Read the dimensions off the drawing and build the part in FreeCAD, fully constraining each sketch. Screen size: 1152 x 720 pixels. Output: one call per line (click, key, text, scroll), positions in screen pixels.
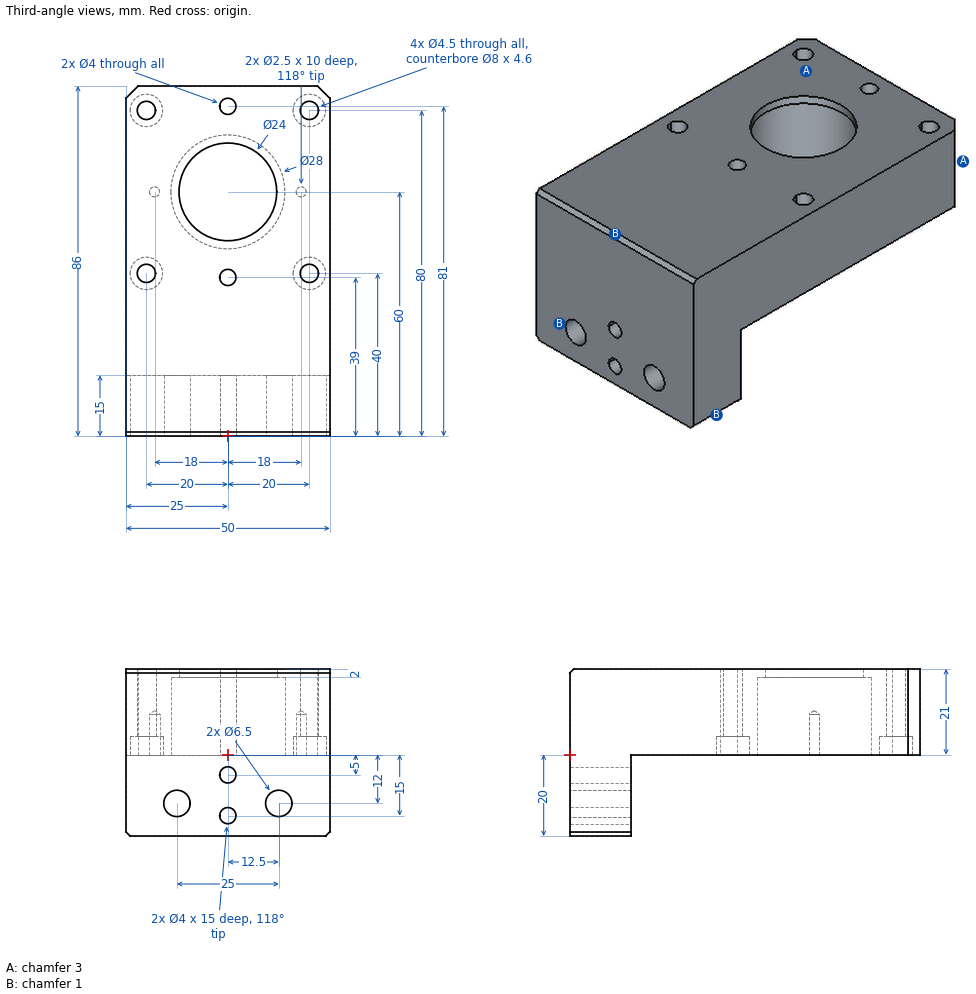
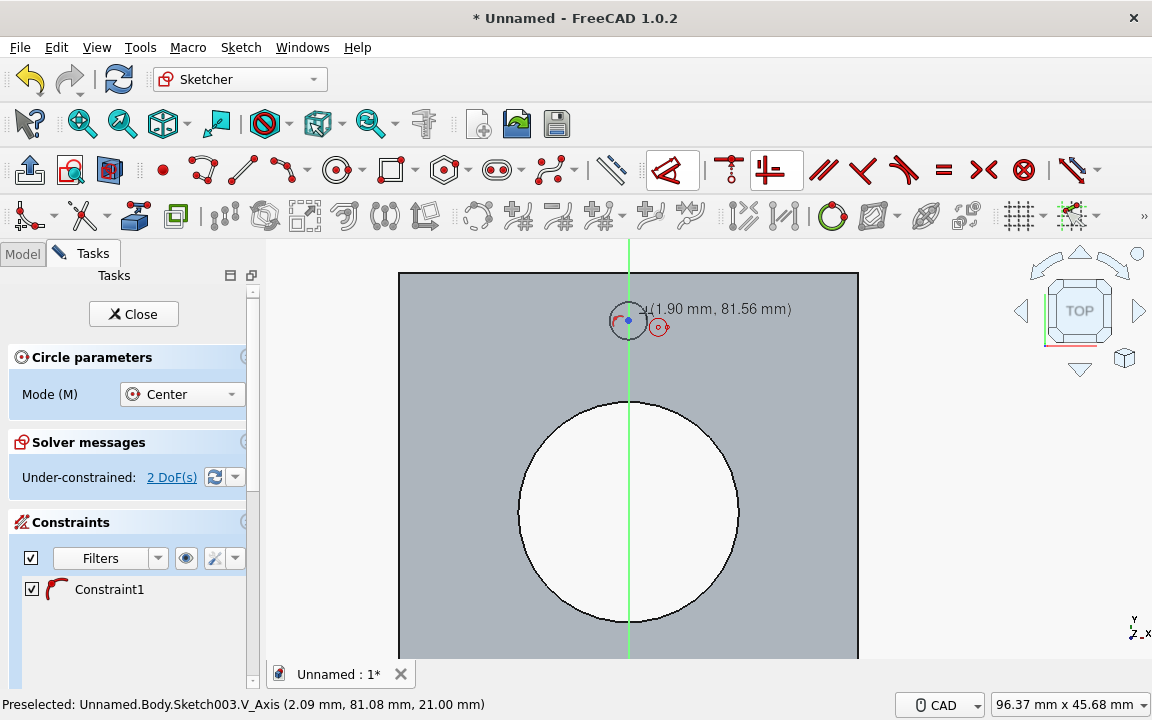
scroll(647, 313, down, 5)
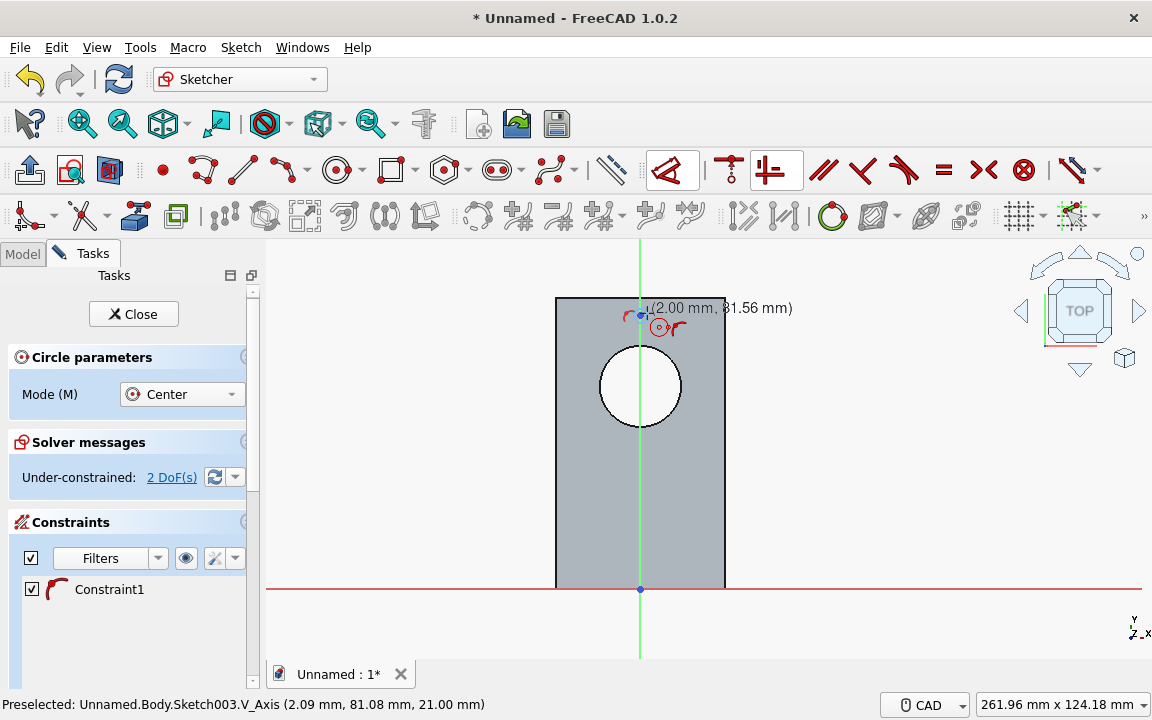
scroll(640, 457, up, 7)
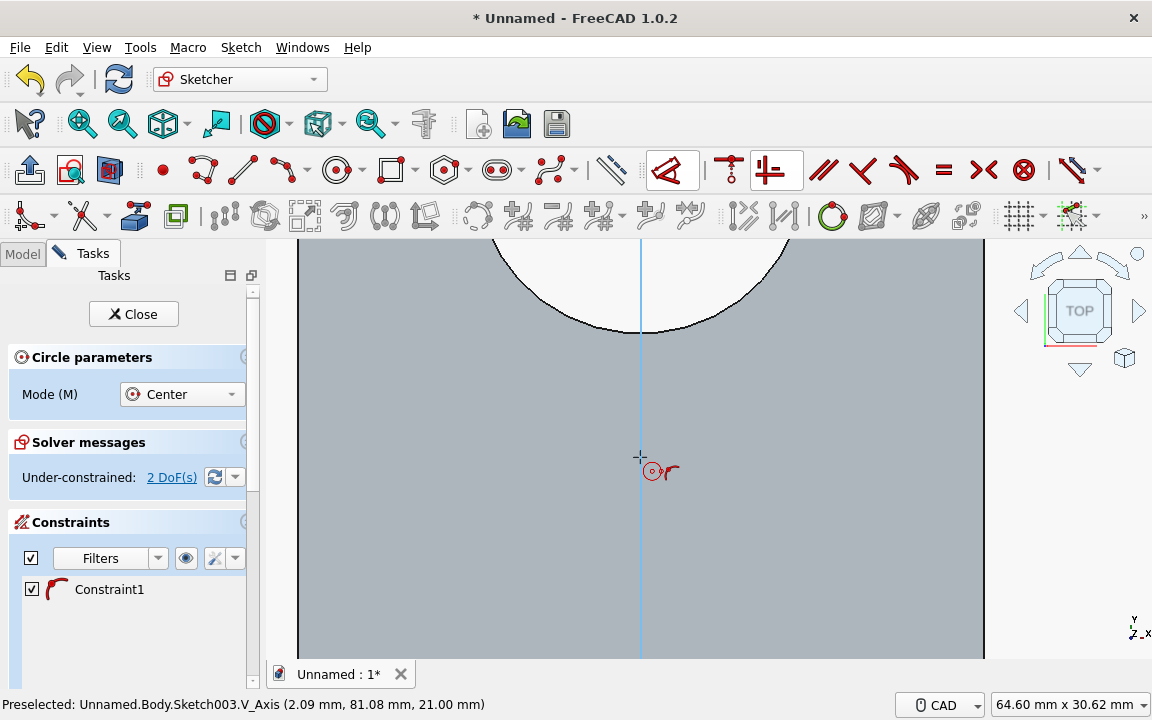
scroll(640, 458, down, 7)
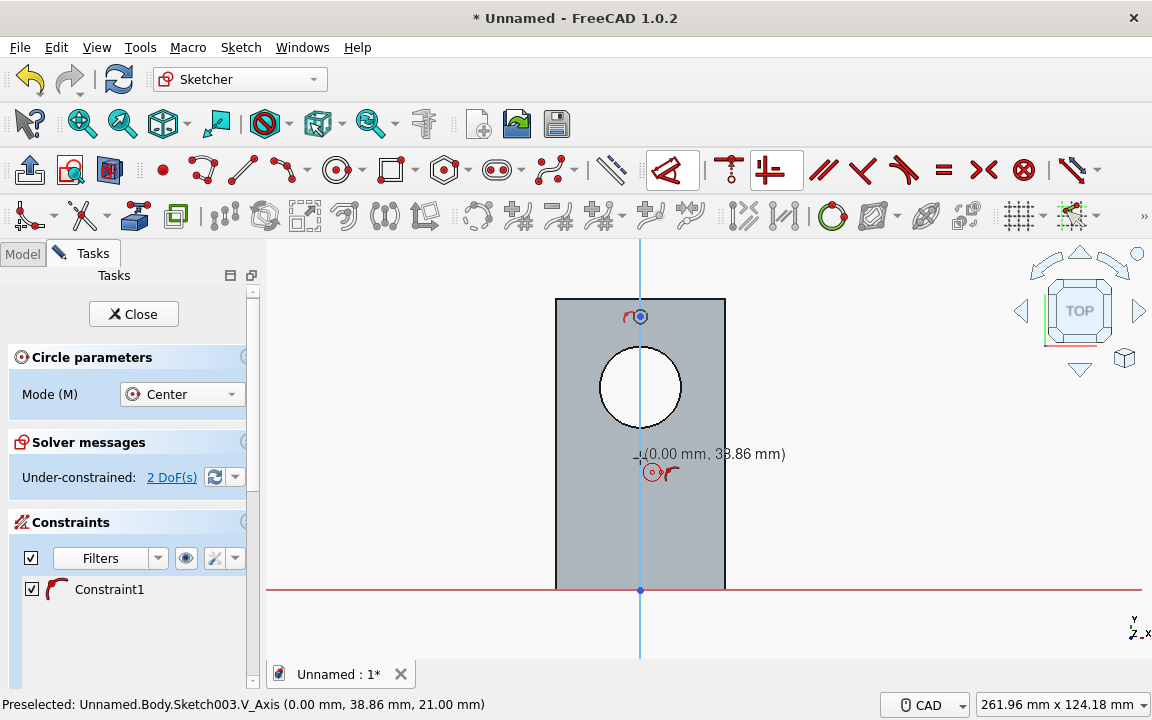
click(640, 458)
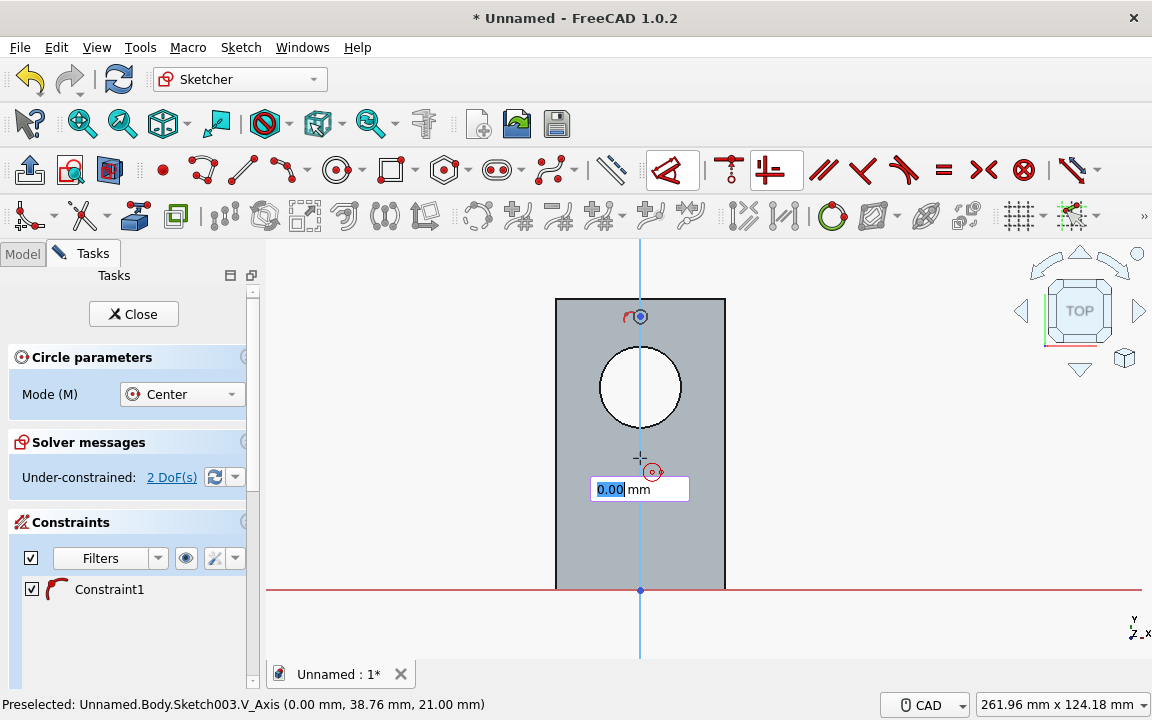
scroll(647, 456, up, 5)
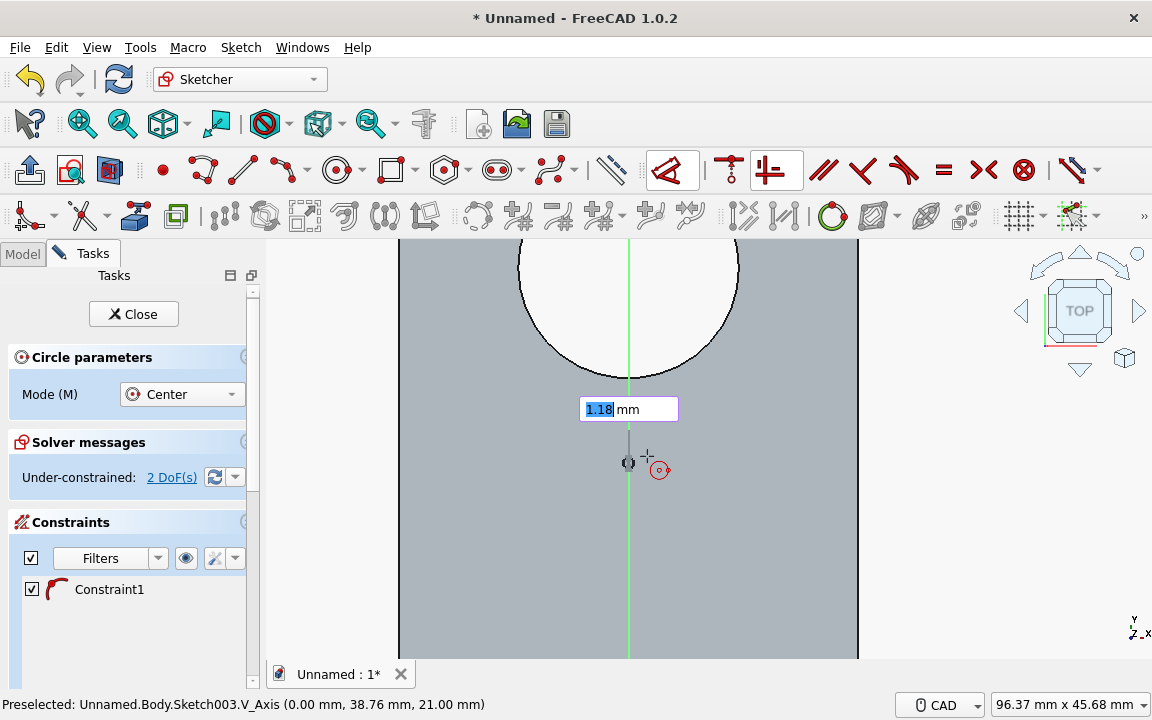
click(646, 455)
key(Escape)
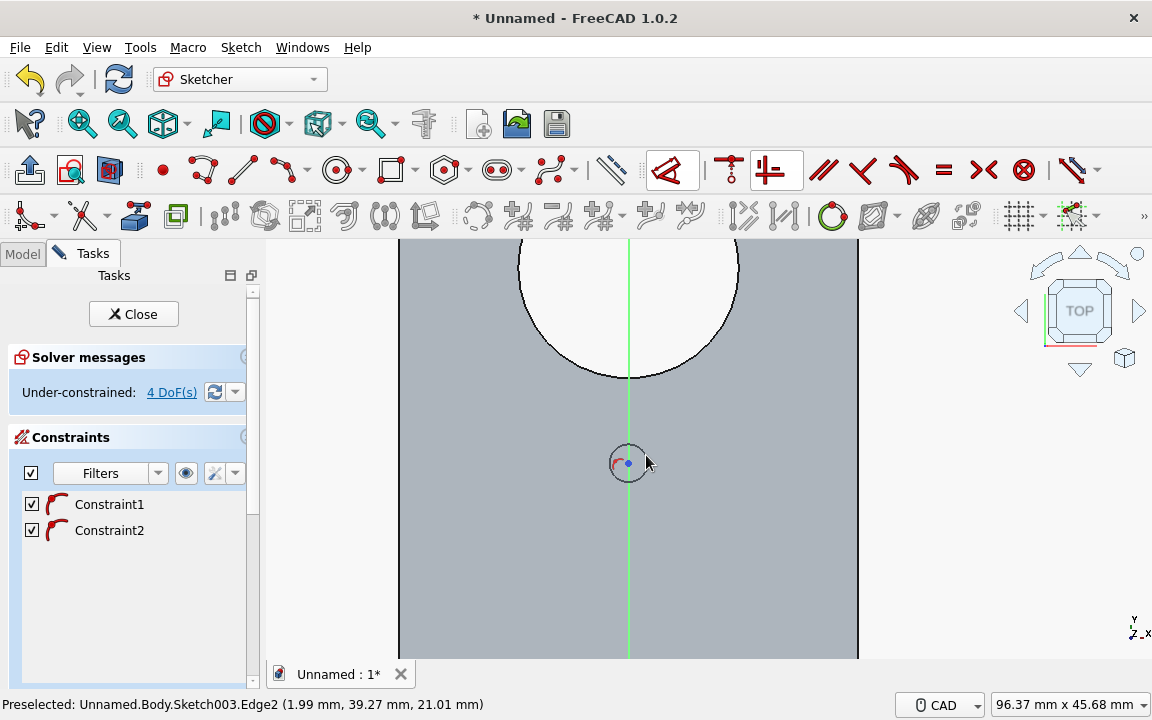
scroll(647, 455, down, 5)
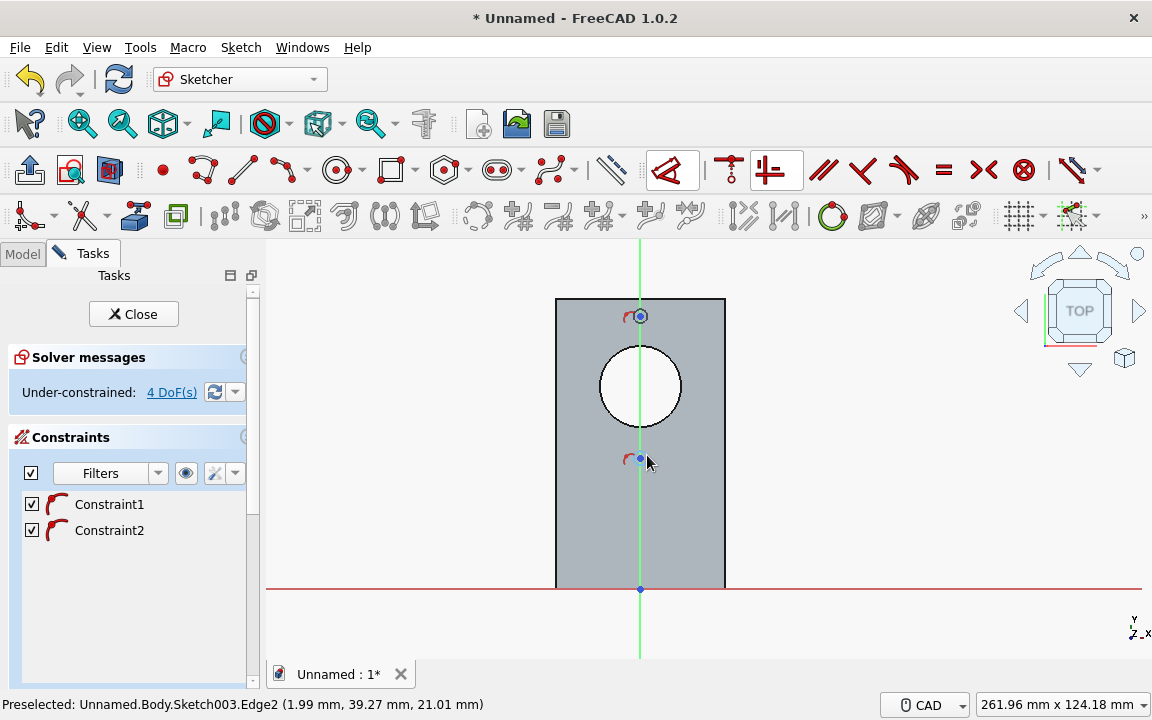
scroll(645, 311, up, 6)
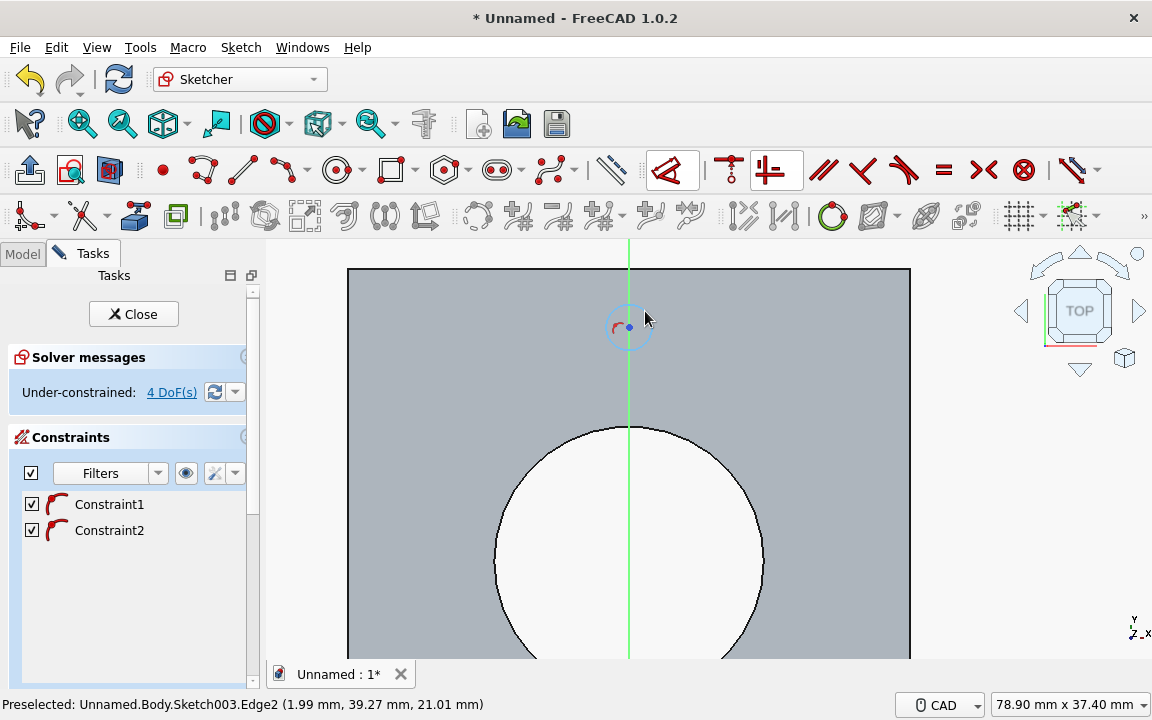
click(645, 311)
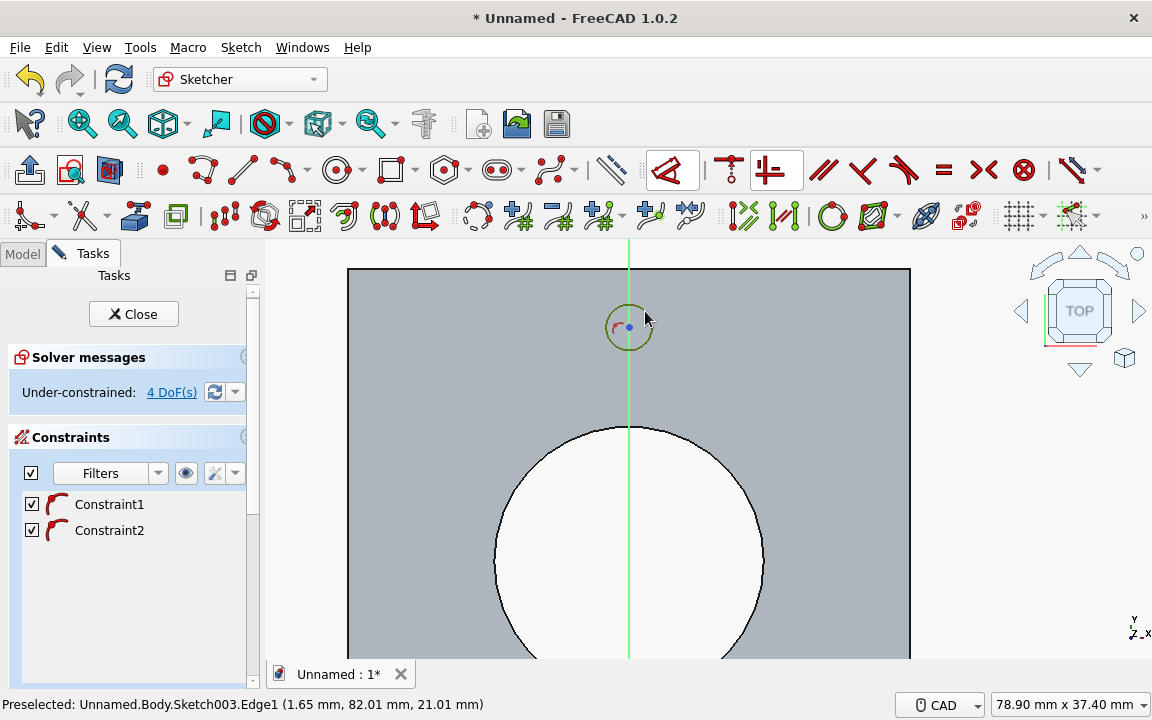
scroll(645, 311, down, 6)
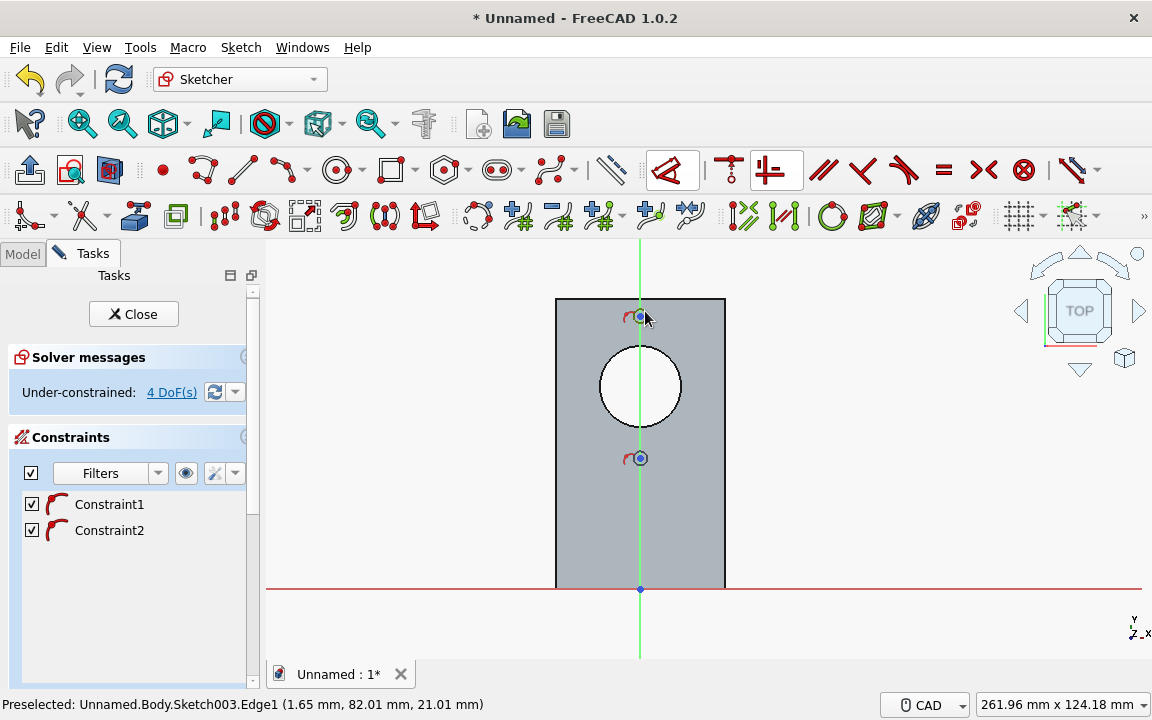
scroll(645, 453, up, 6)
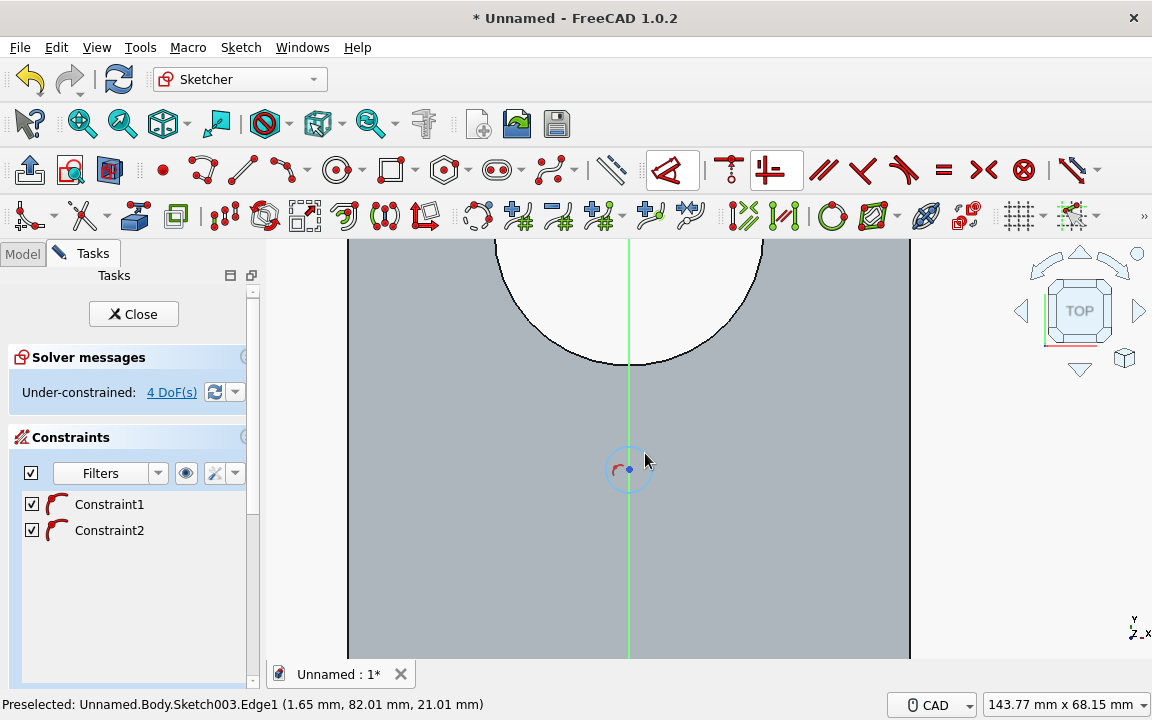
click(645, 453)